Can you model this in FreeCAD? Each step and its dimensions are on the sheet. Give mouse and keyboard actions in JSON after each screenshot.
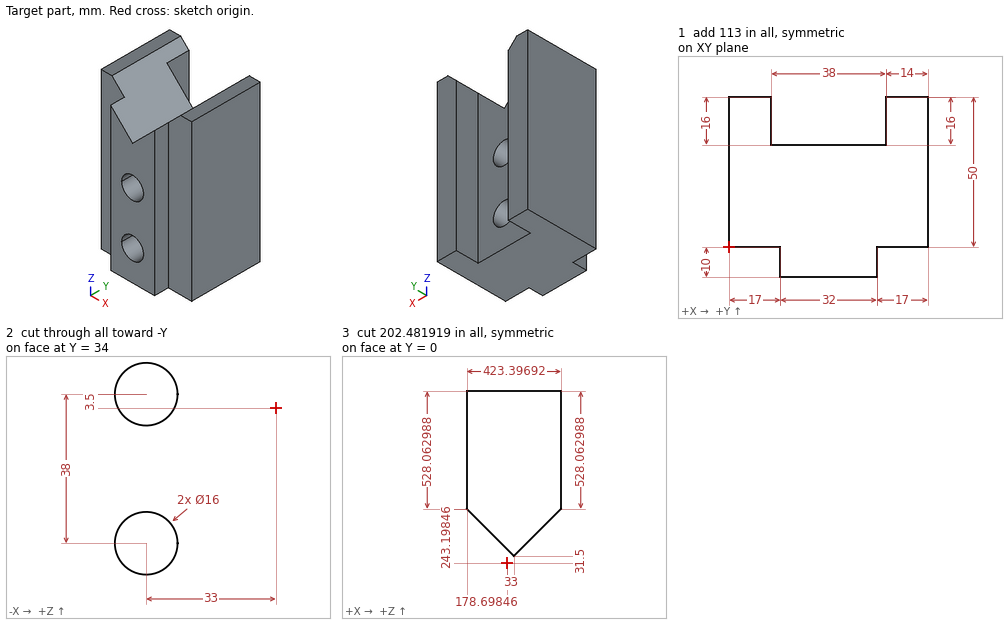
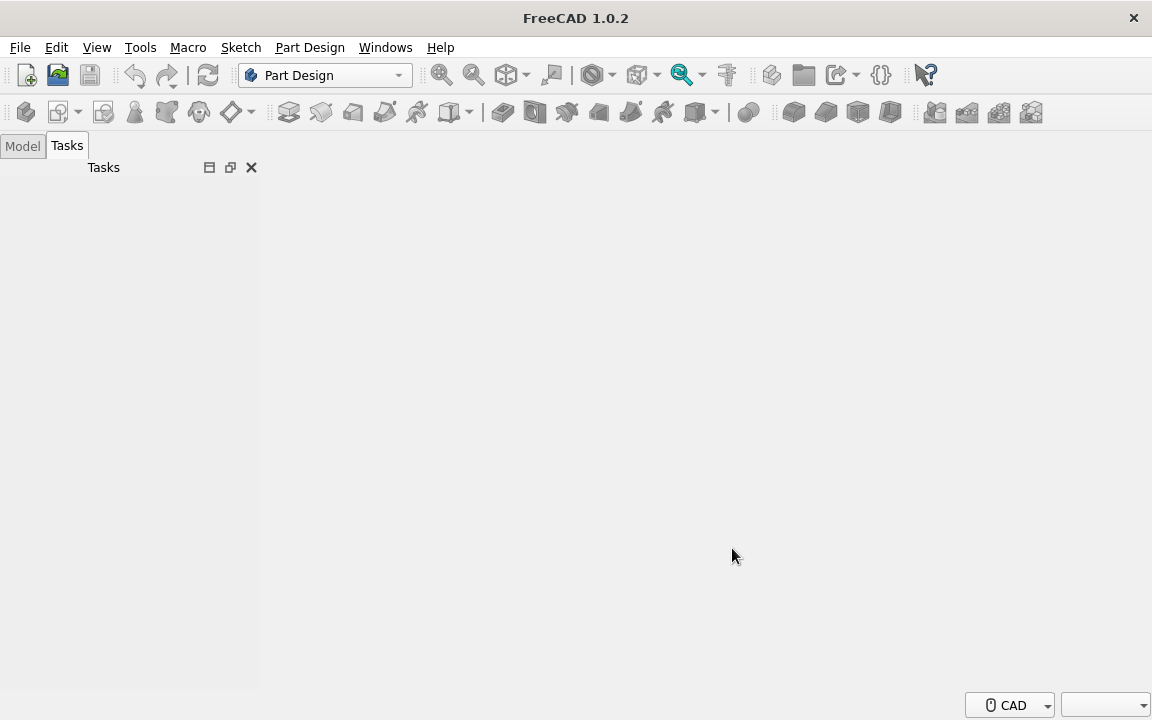
{"action": "left_click", "coordinate": [26, 76]}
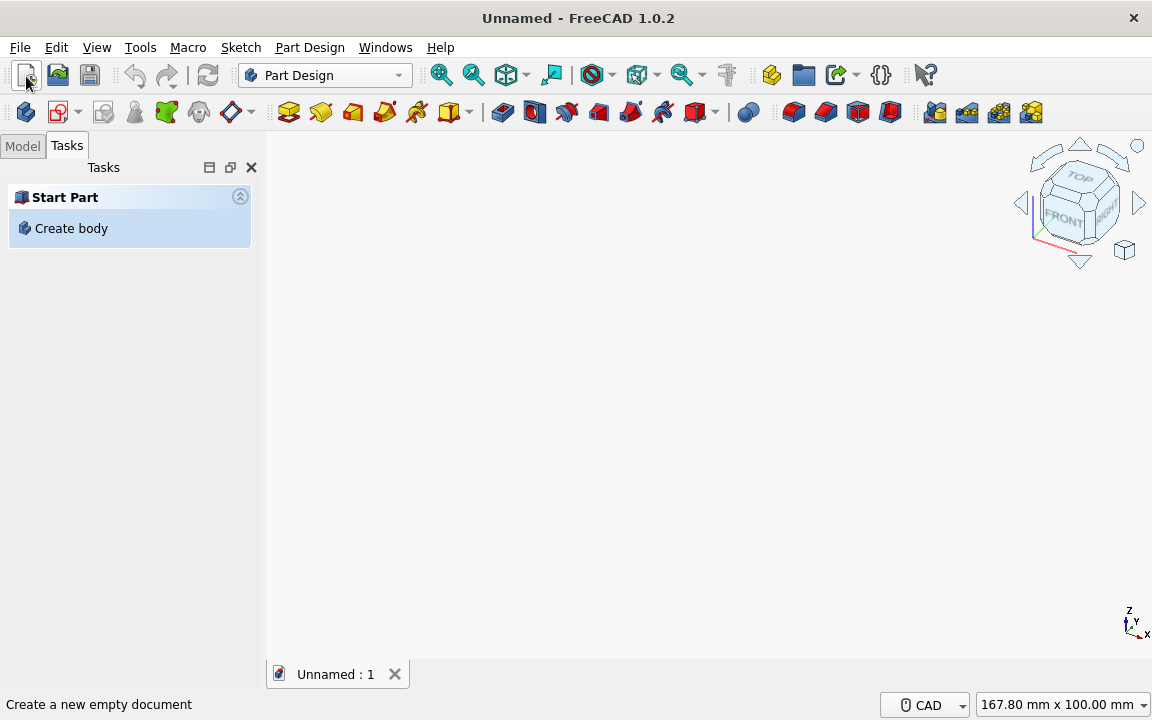
{"action": "left_click", "coordinate": [58, 112]}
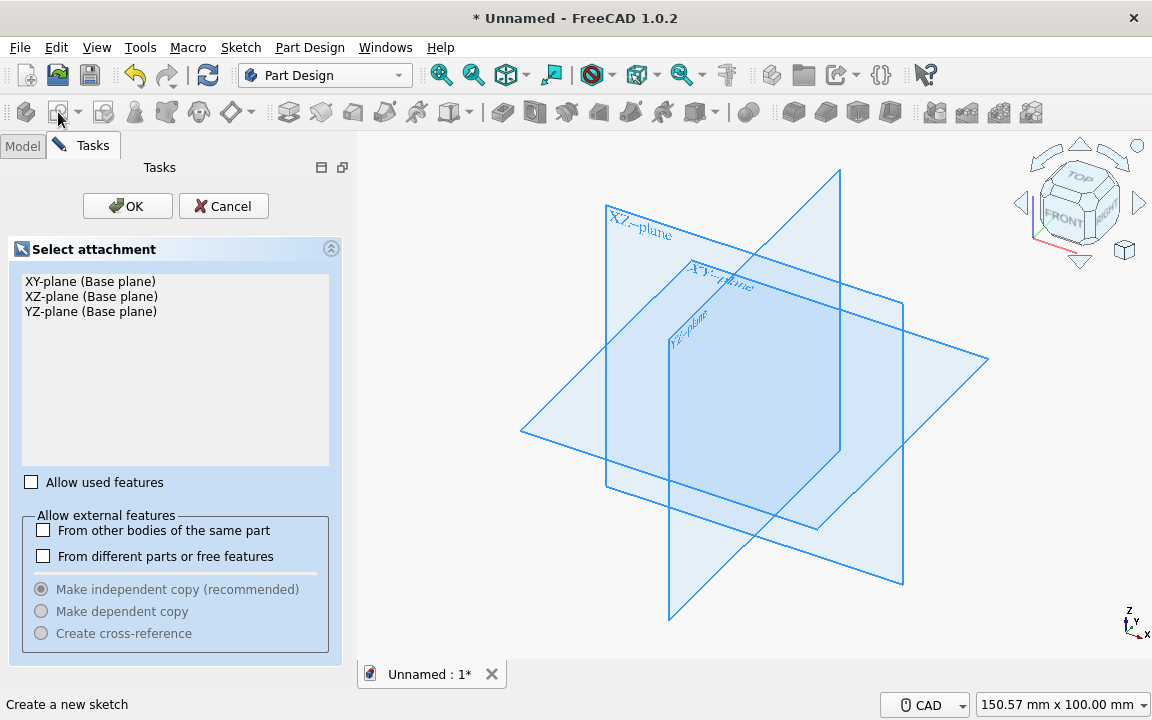
{"action": "left_click", "coordinate": [82, 282]}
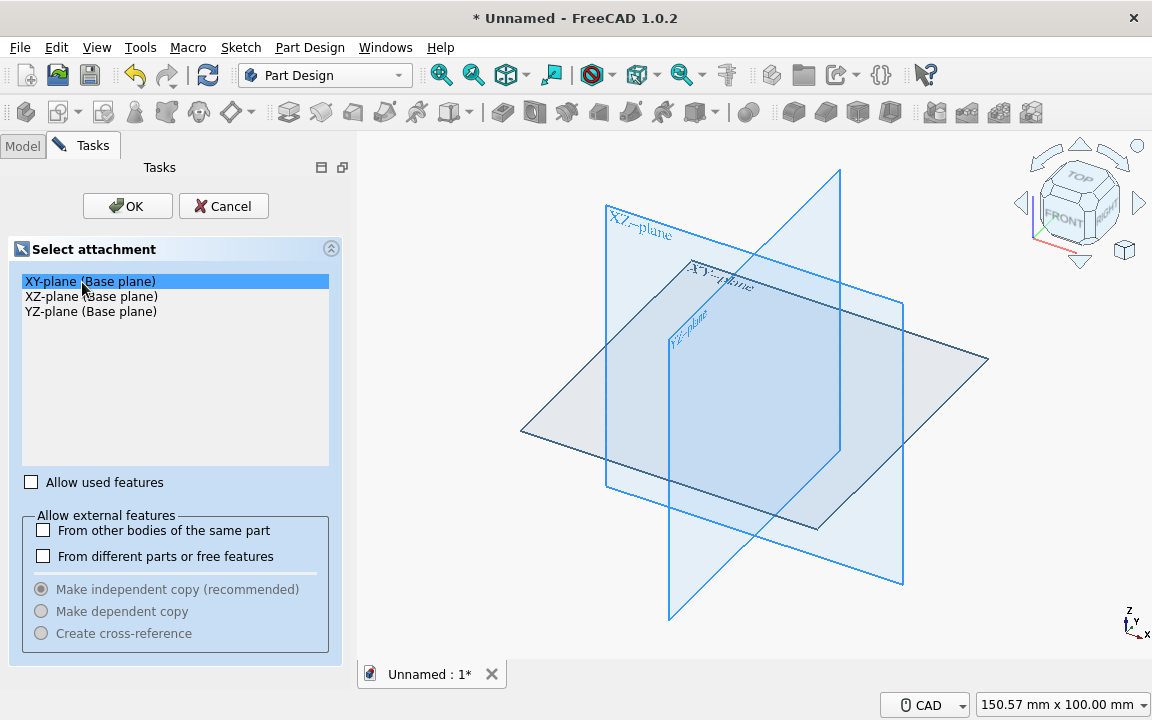
{"action": "left_click", "coordinate": [128, 206]}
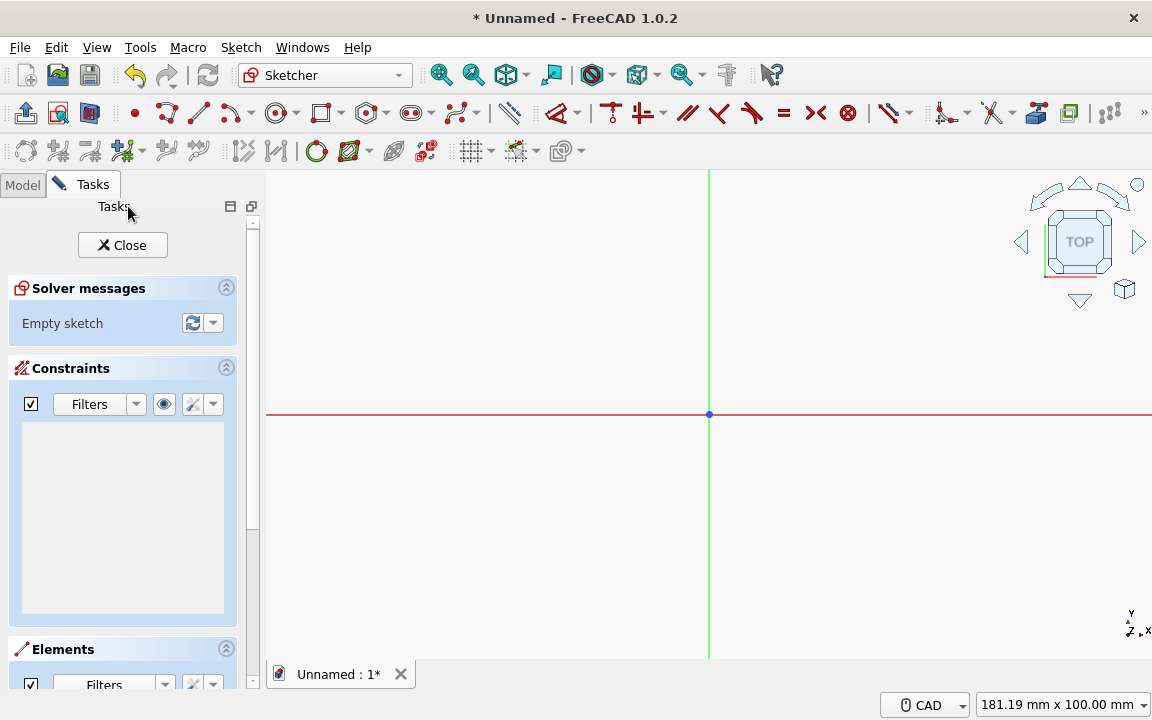
{"action": "scroll", "coordinate": [294, 631], "scroll_direction": "down", "scroll_amount": 1}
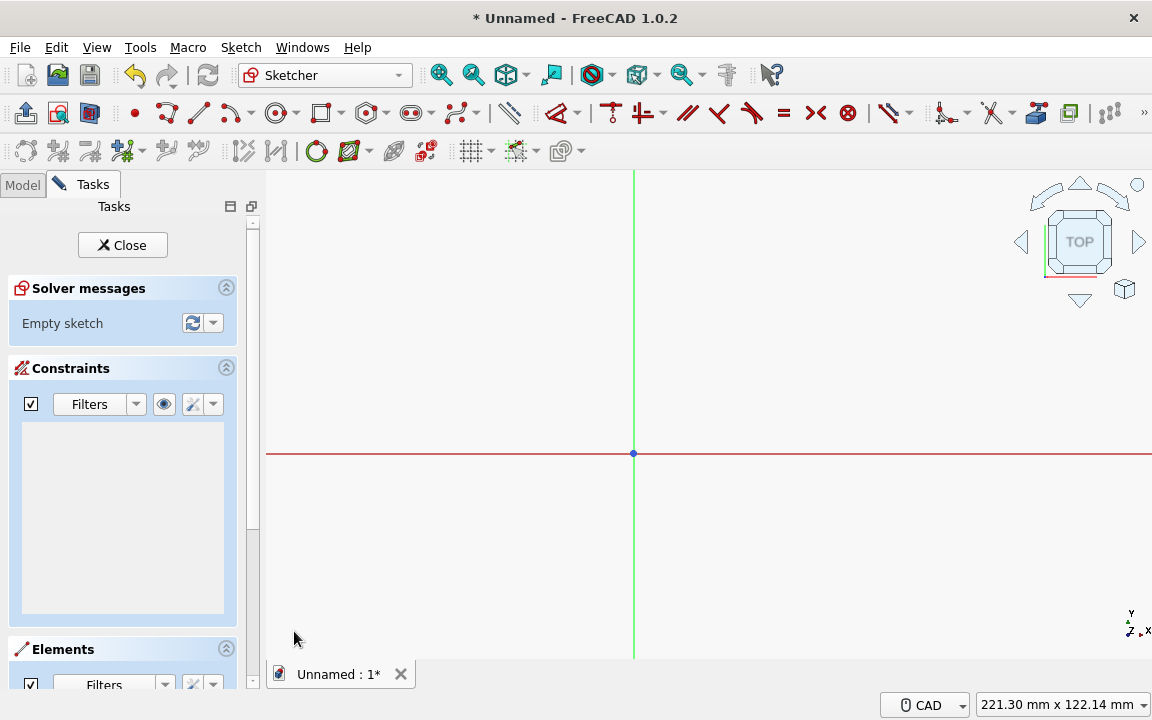
{"action": "left_click", "coordinate": [168, 114]}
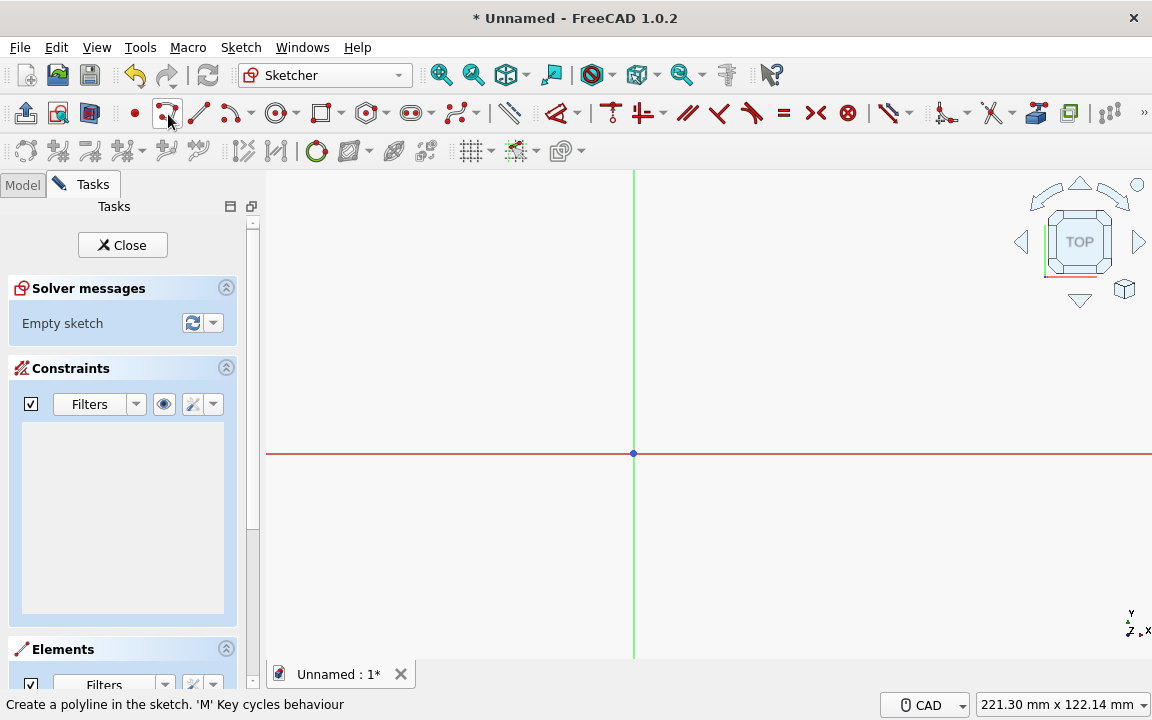
{"action": "left_click", "coordinate": [634, 454]}
{"action": "left_click", "coordinate": [702, 445]}
{"action": "left_click", "coordinate": [702, 494]}
{"action": "left_click", "coordinate": [830, 494]}
{"action": "left_click", "coordinate": [830, 454]}
{"action": "left_click", "coordinate": [898, 445]}
{"action": "left_click", "coordinate": [898, 254]}
{"action": "left_click", "coordinate": [842, 254]}
{"action": "left_click", "coordinate": [842, 318]}
{"action": "left_click", "coordinate": [690, 318]}
{"action": "left_click", "coordinate": [690, 254]}
{"action": "left_click", "coordinate": [643, 254]}
{"action": "left_click", "coordinate": [634, 454]}
{"action": "key", "text": "Escape"}
{"action": "key", "text": "Escape"}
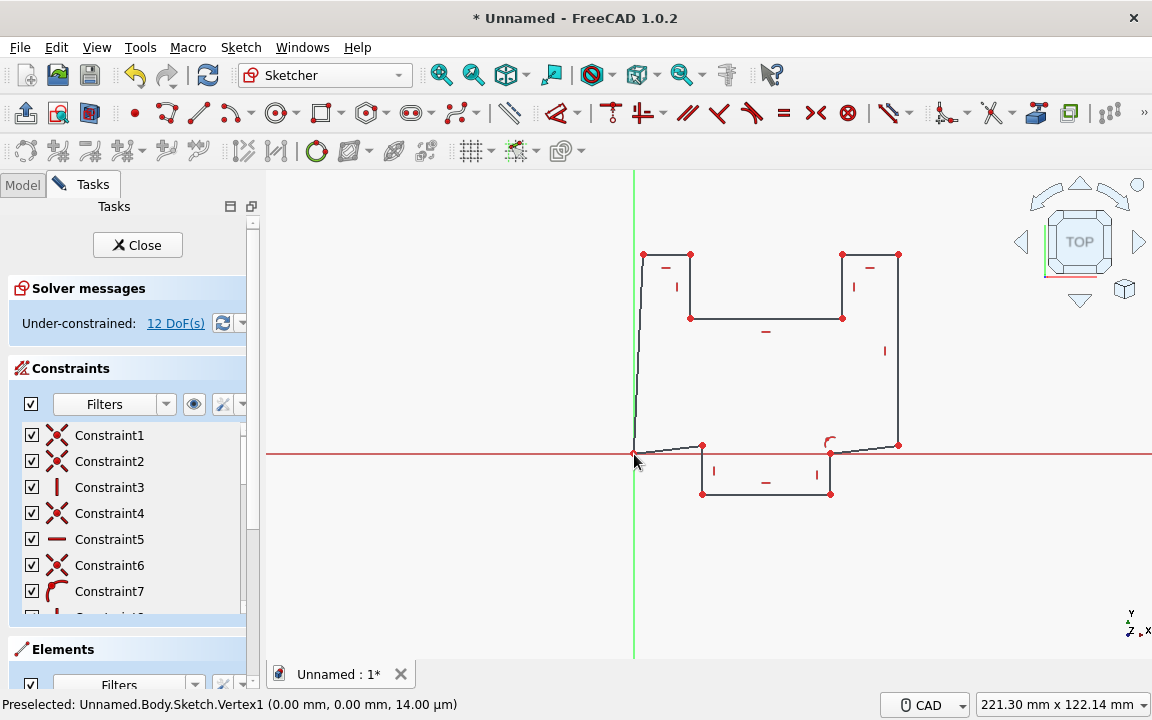
{"action": "left_click", "coordinate": [654, 452]}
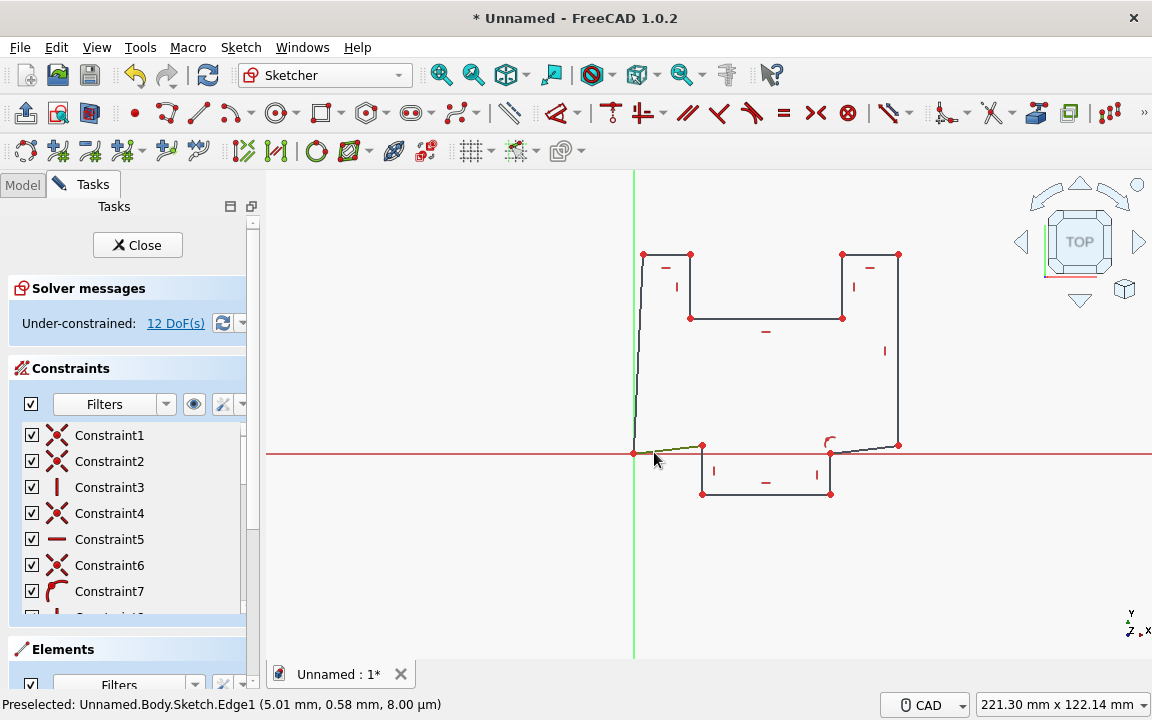
{"action": "key", "text": "h"}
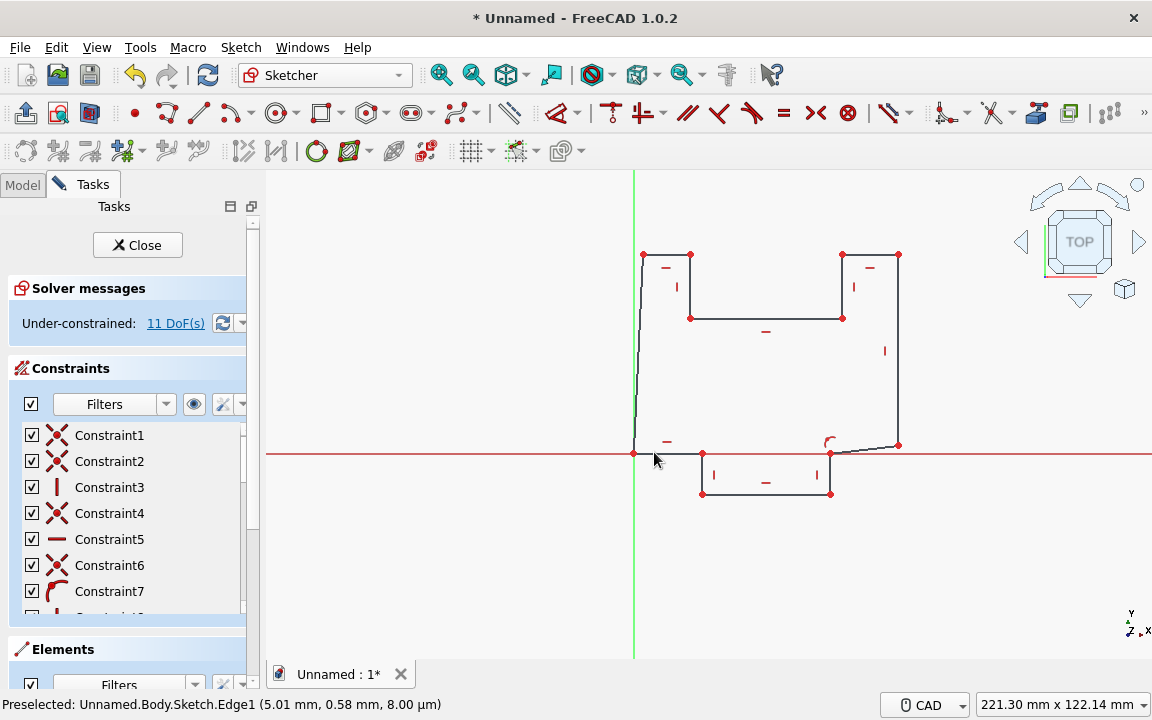
{"action": "left_click", "coordinate": [850, 452]}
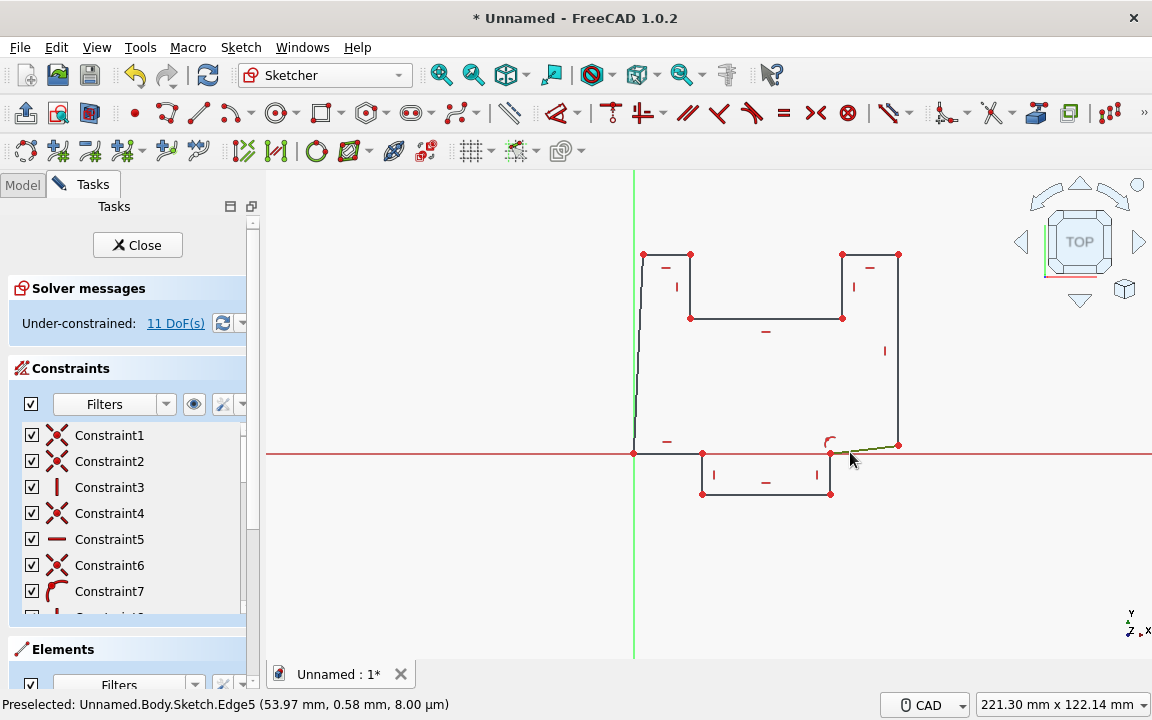
{"action": "left_click", "coordinate": [666, 114]}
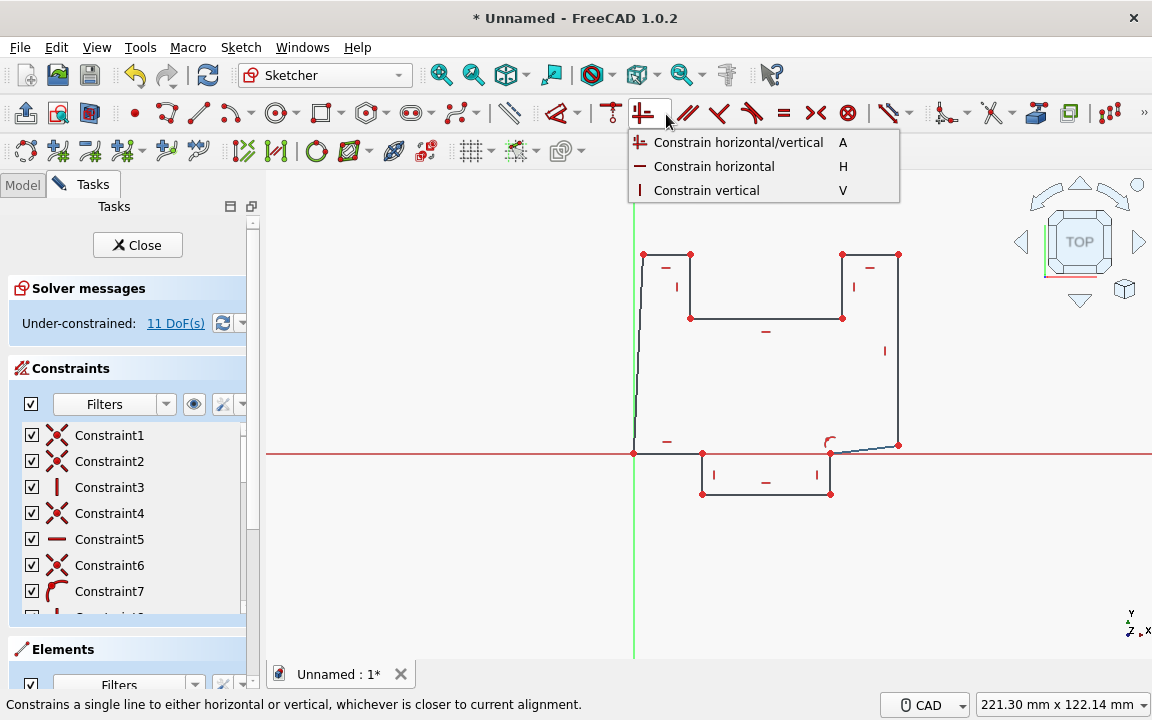
{"action": "left_click", "coordinate": [764, 166]}